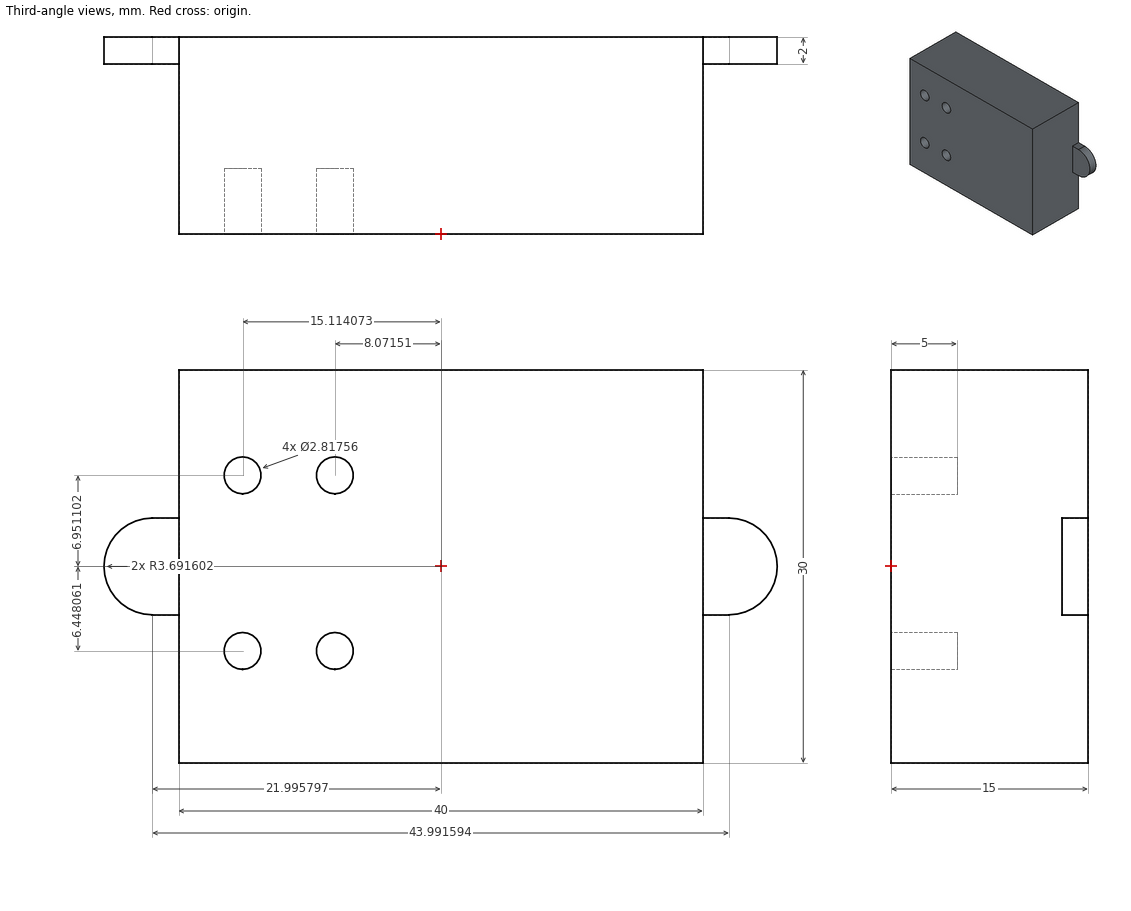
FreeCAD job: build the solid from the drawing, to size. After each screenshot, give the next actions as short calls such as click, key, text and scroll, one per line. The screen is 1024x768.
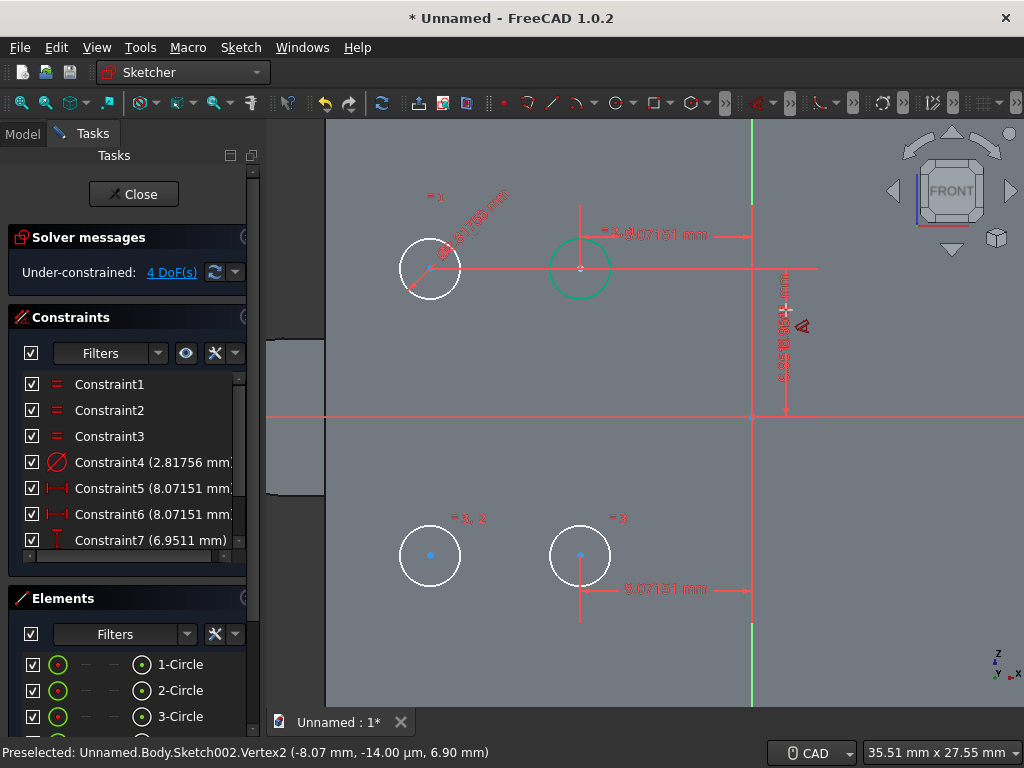
click(430, 556)
click(786, 487)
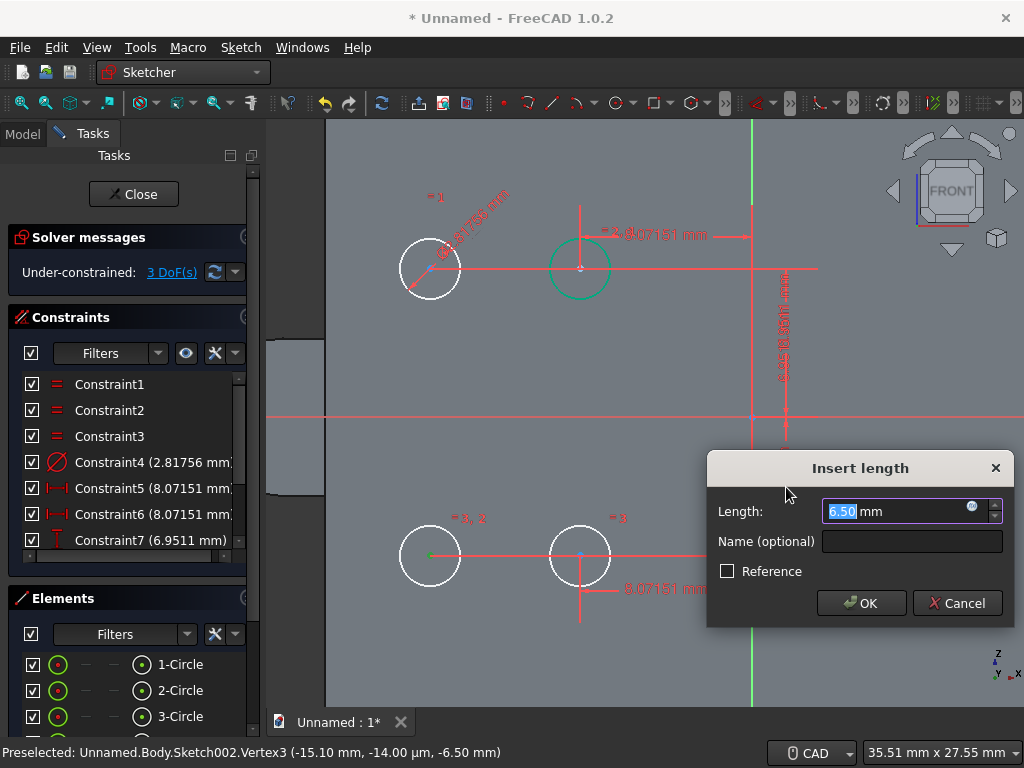
text(6.448061)
key(Return)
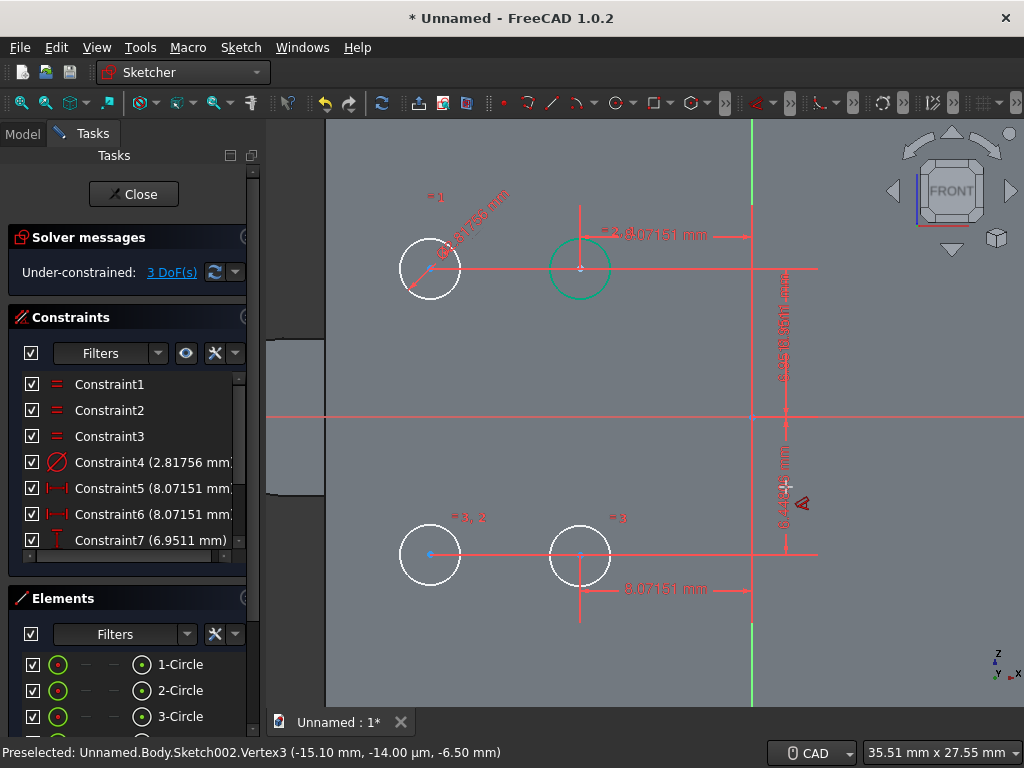
click(580, 556)
click(786, 455)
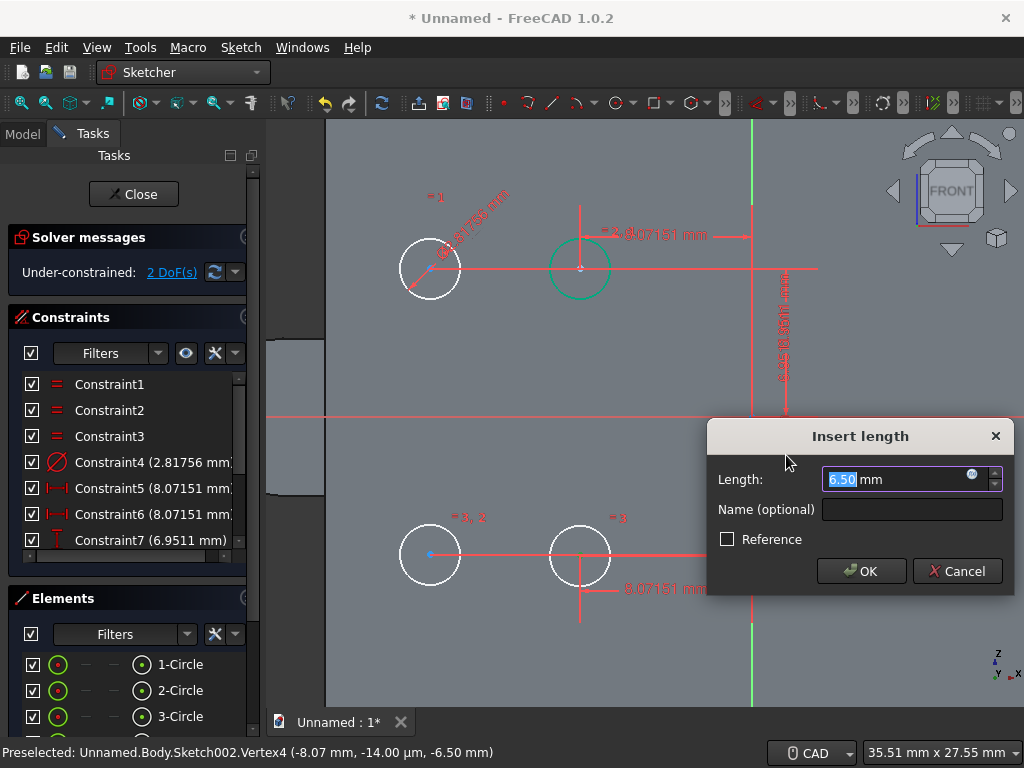
text(6.448061)
key(Return)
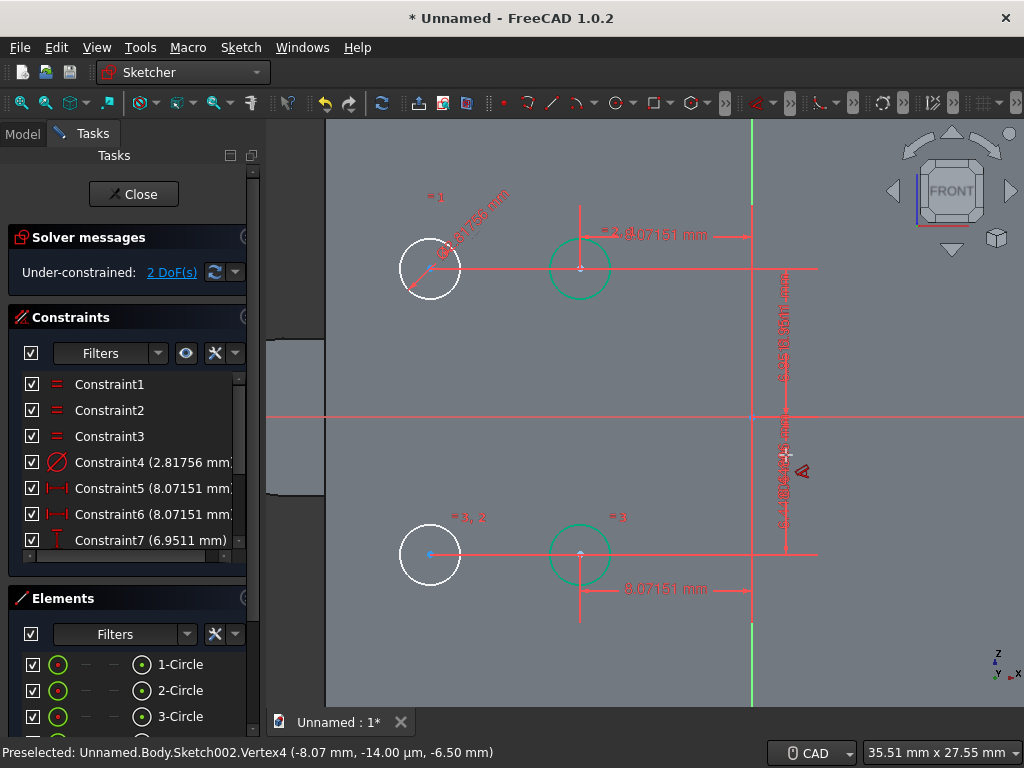
click(430, 269)
click(591, 451)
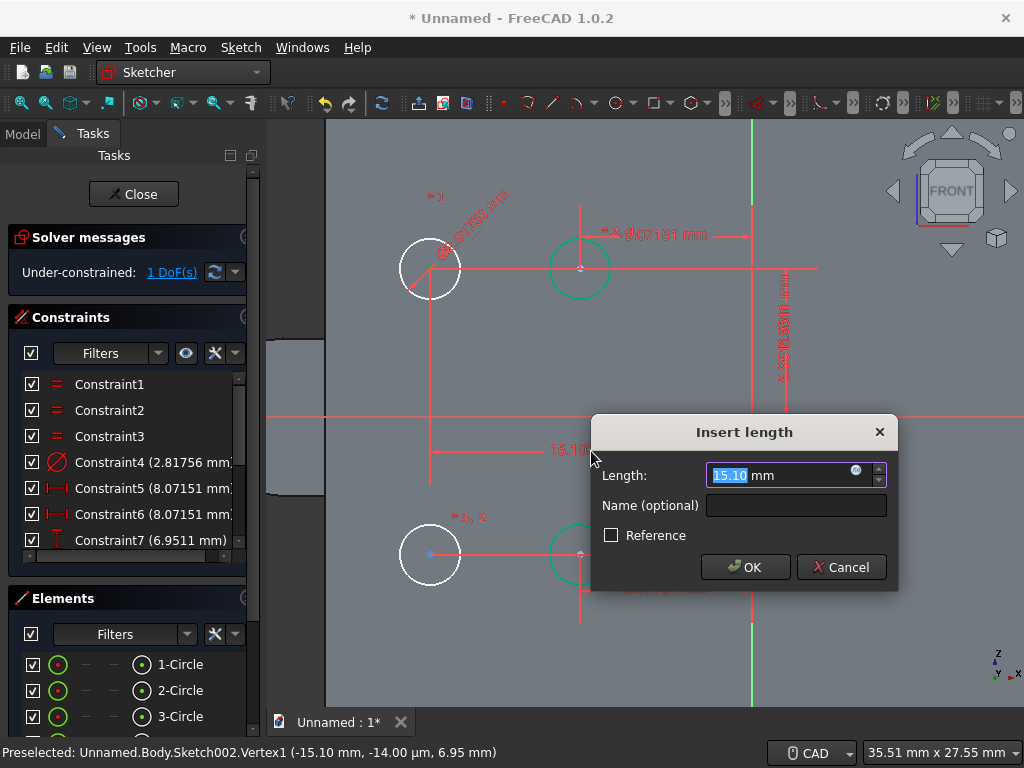
text(15.114073)
key(Return)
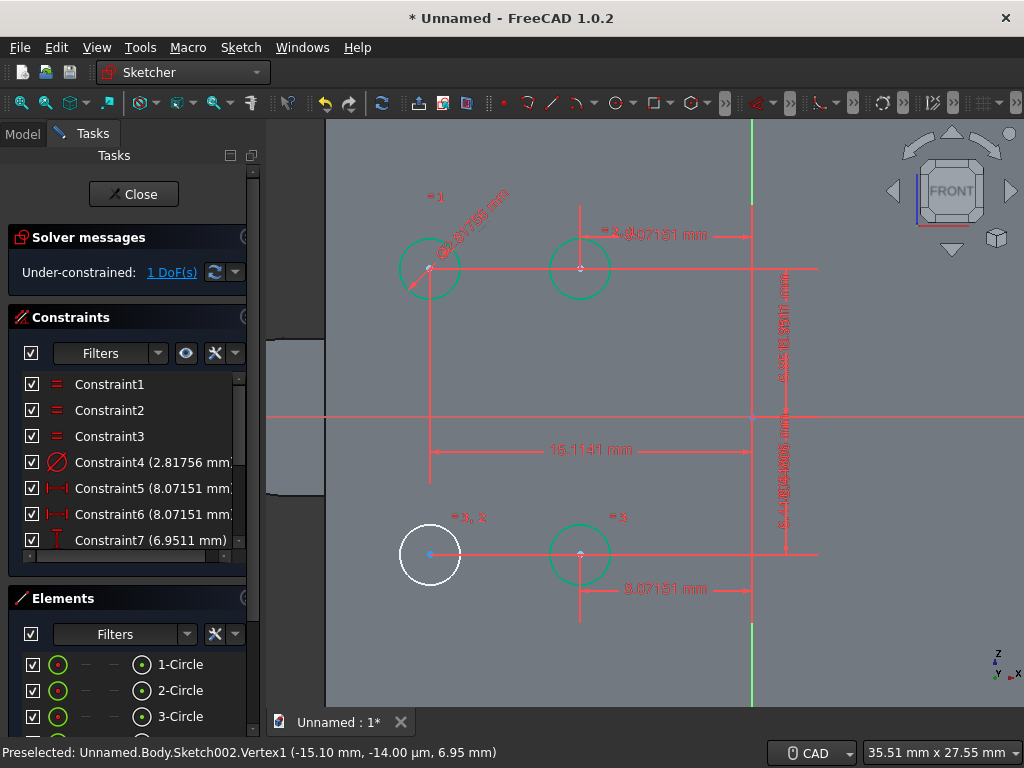
click(430, 555)
click(517, 589)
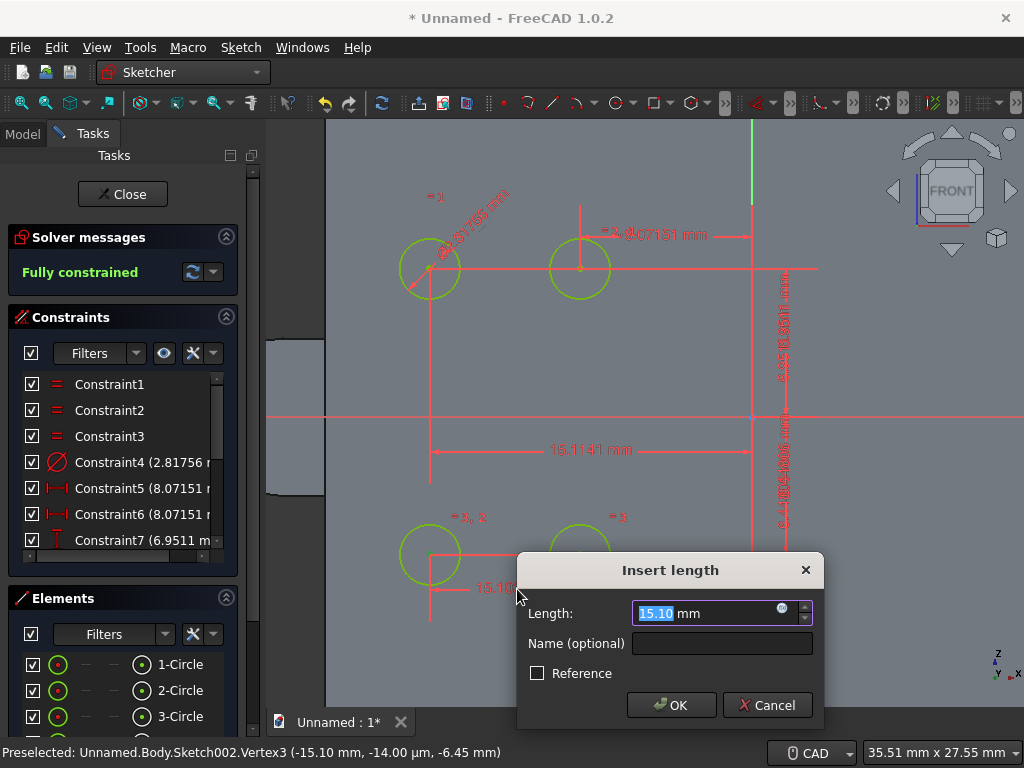
text(15.114073)
key(Return)
key(Escape)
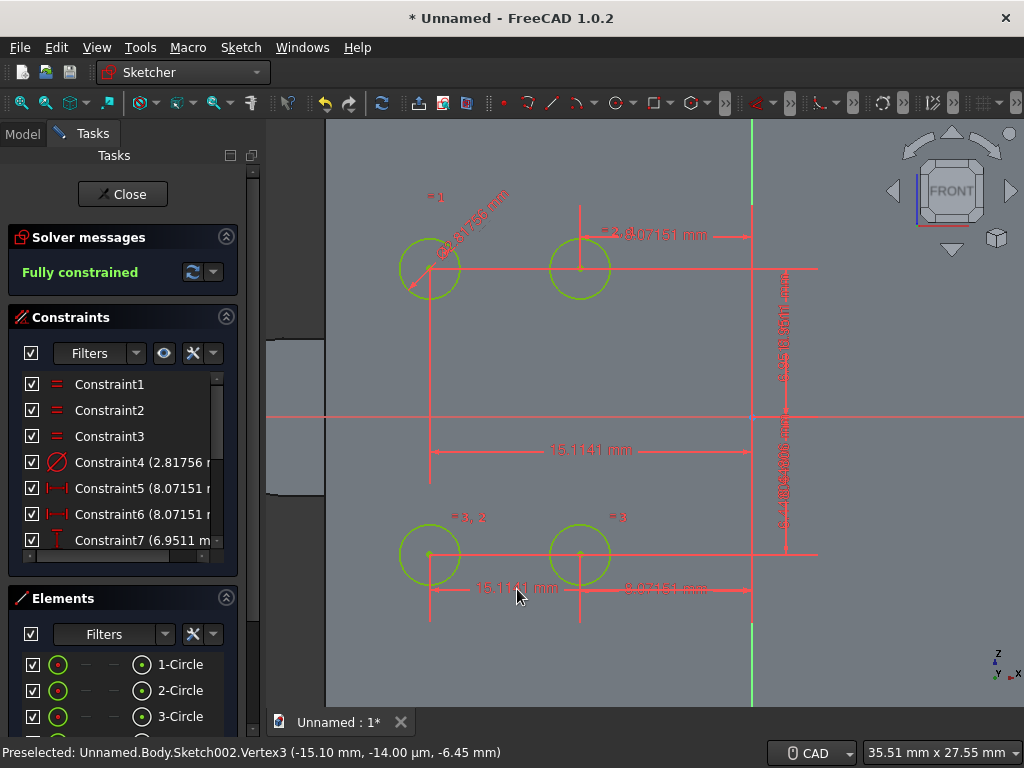
click(123, 194)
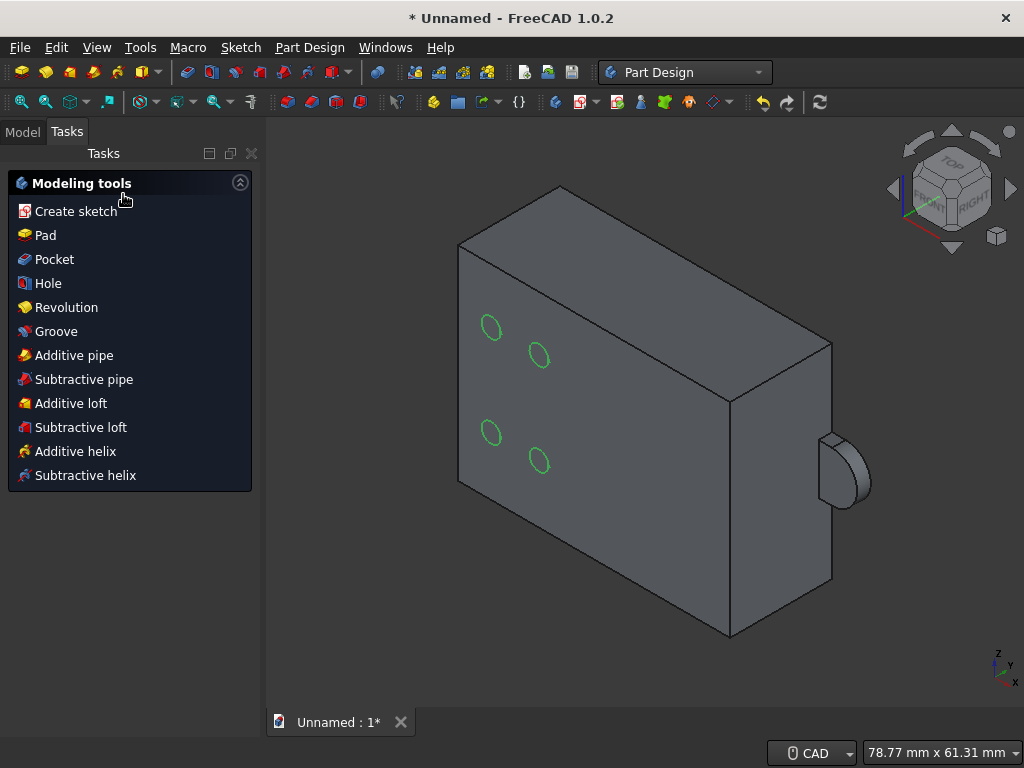
click(188, 72)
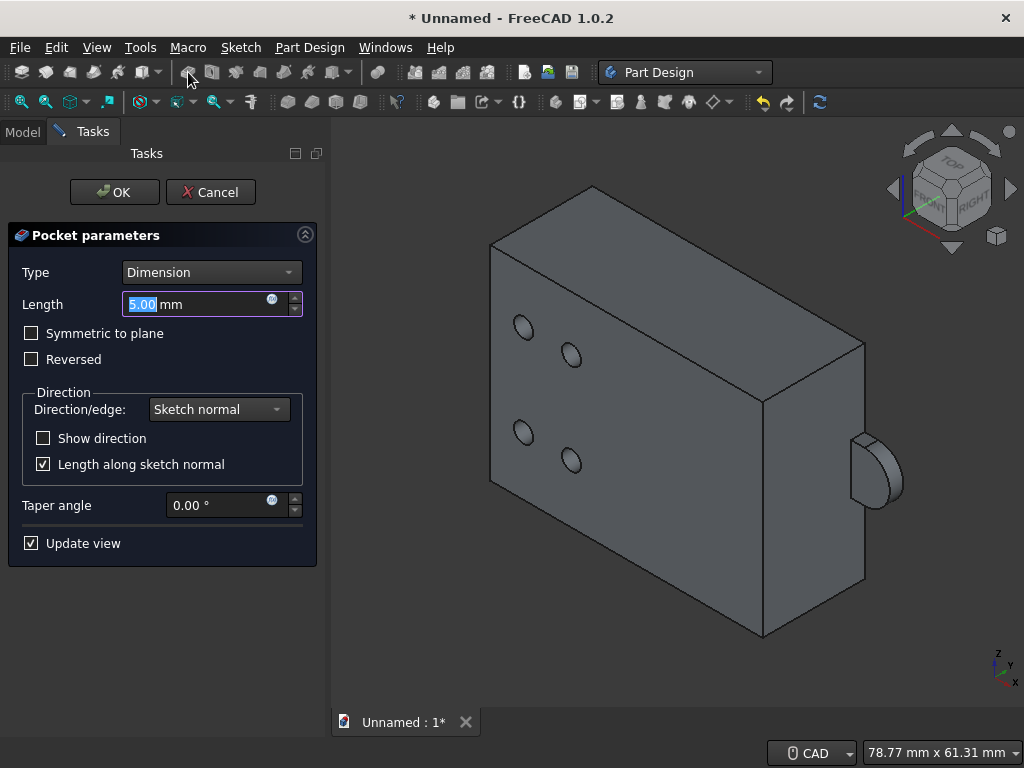
text(5)
key(Tab)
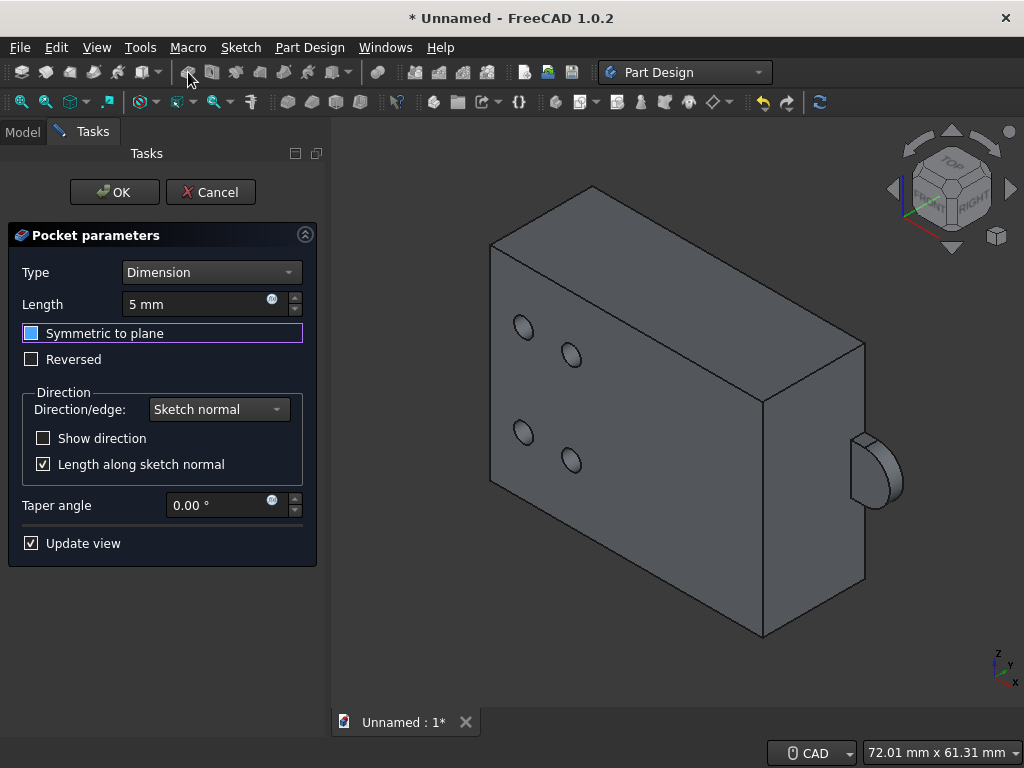
click(115, 192)